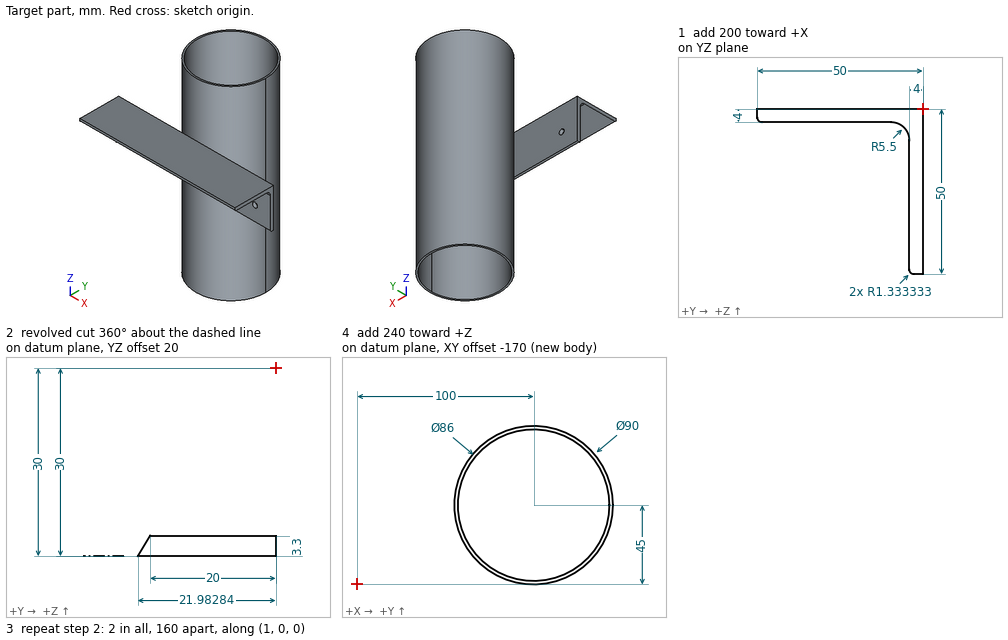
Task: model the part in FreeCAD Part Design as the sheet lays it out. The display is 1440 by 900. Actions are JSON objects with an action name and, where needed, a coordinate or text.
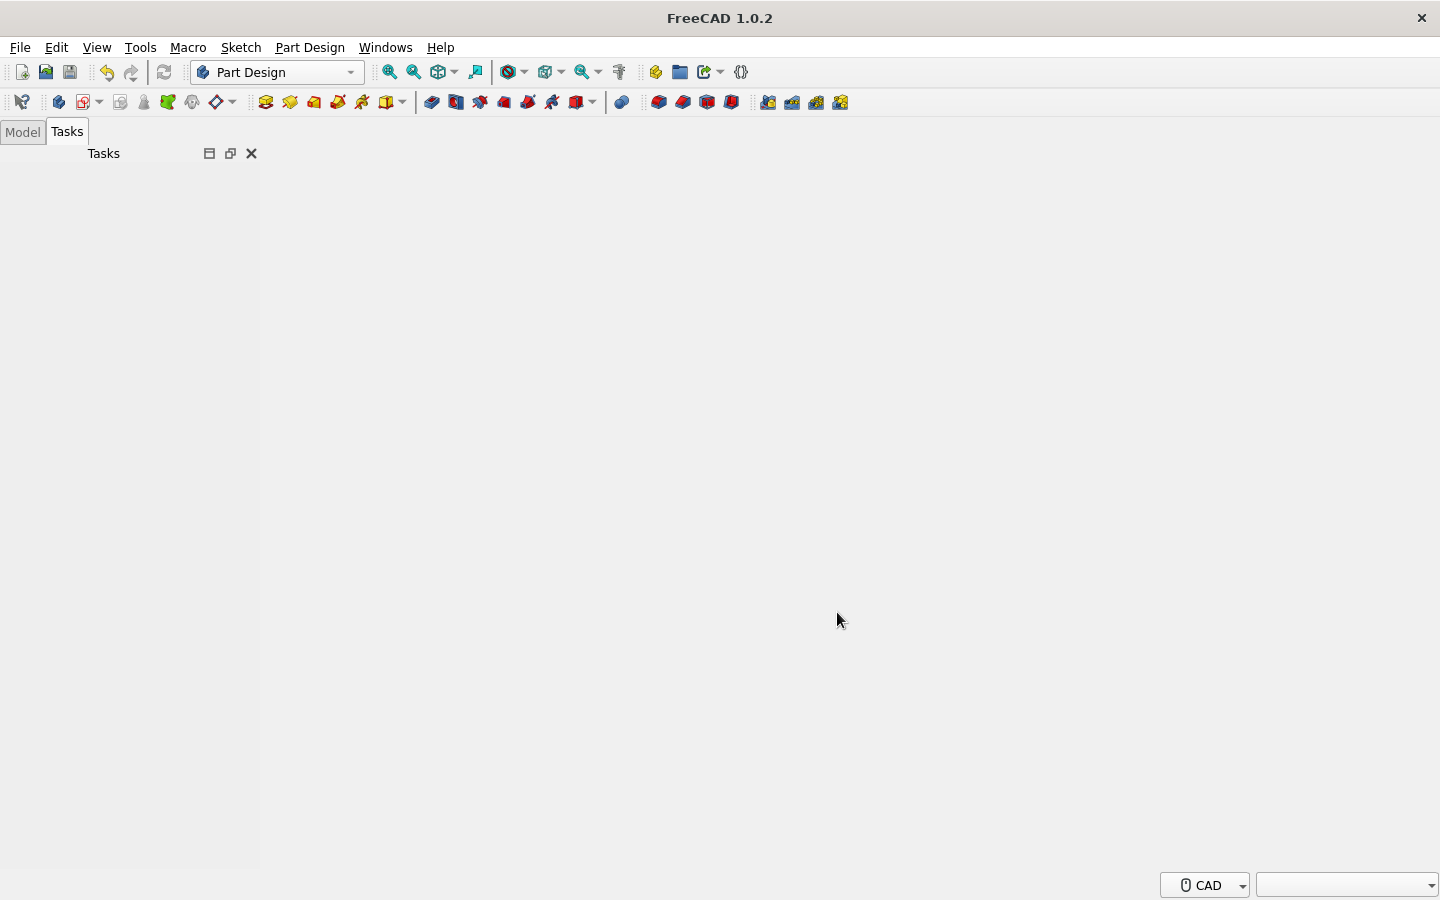
{"action": "left_click", "coordinate": [22, 72]}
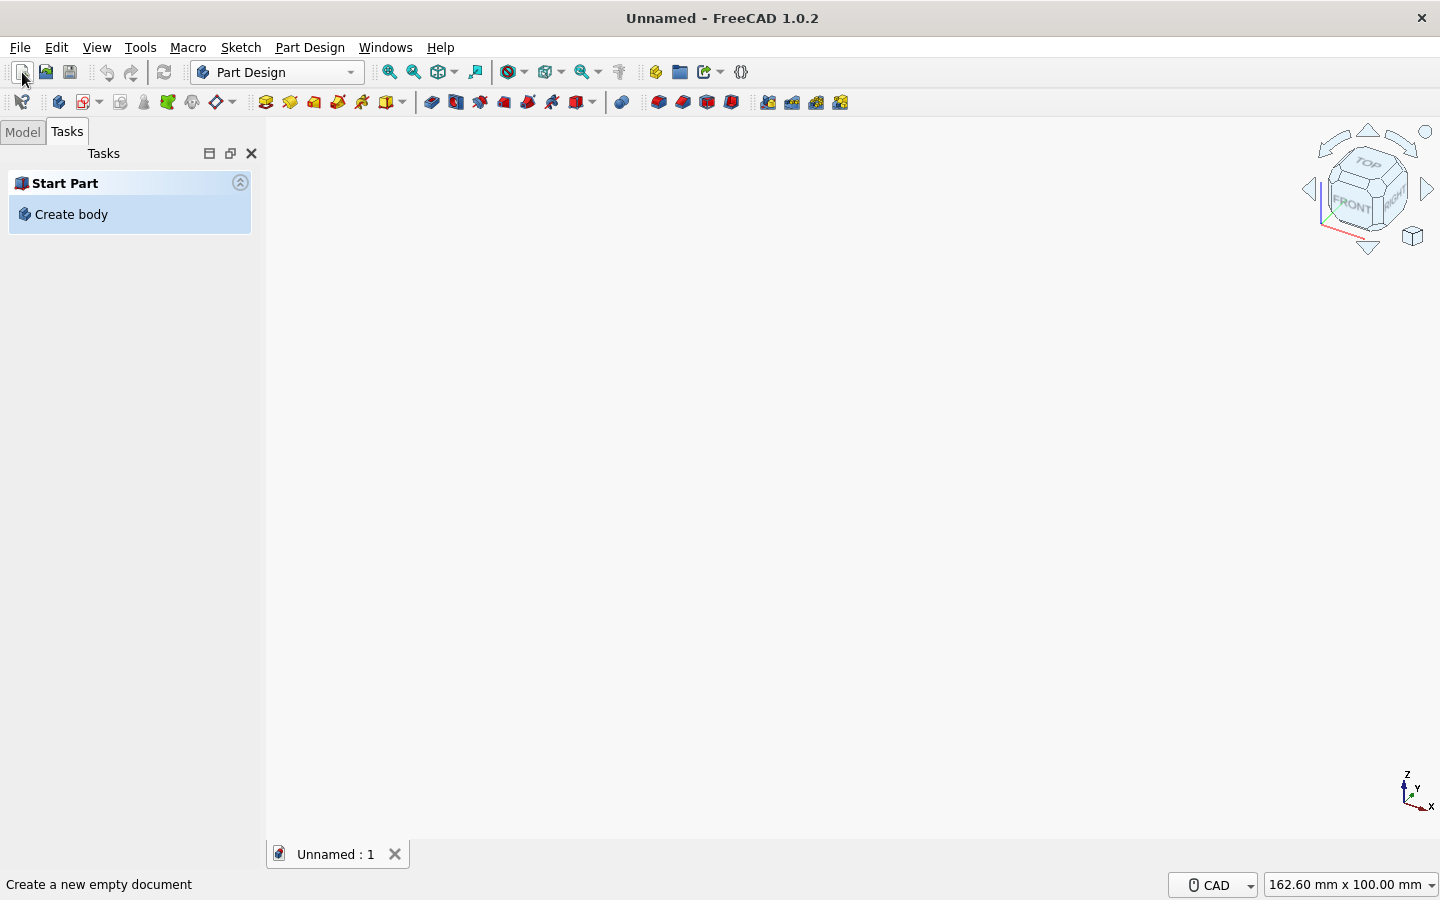
{"action": "left_click", "coordinate": [84, 102]}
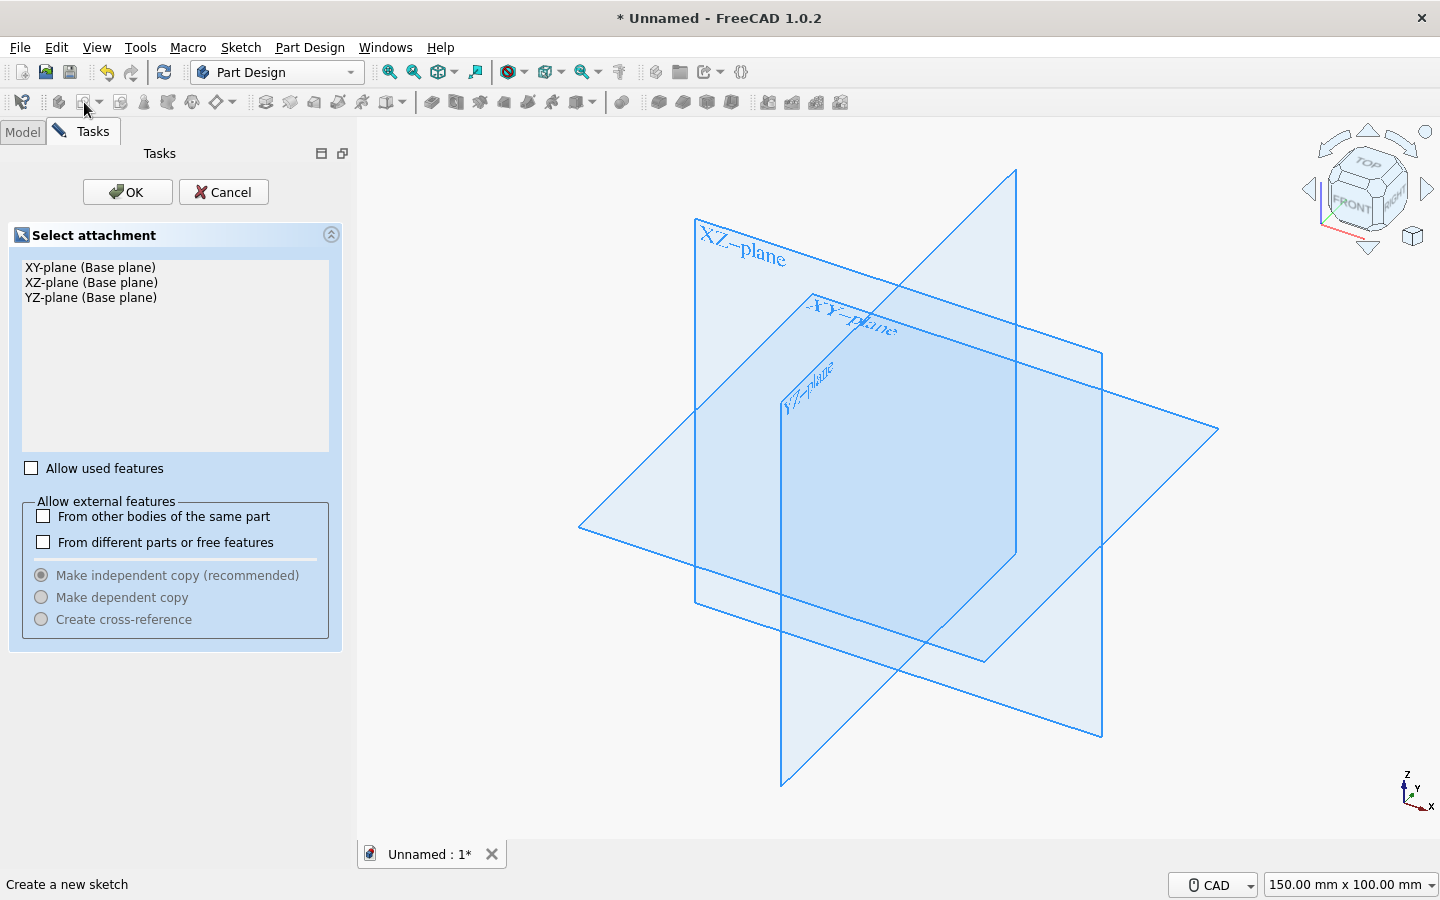
{"action": "left_click", "coordinate": [82, 298]}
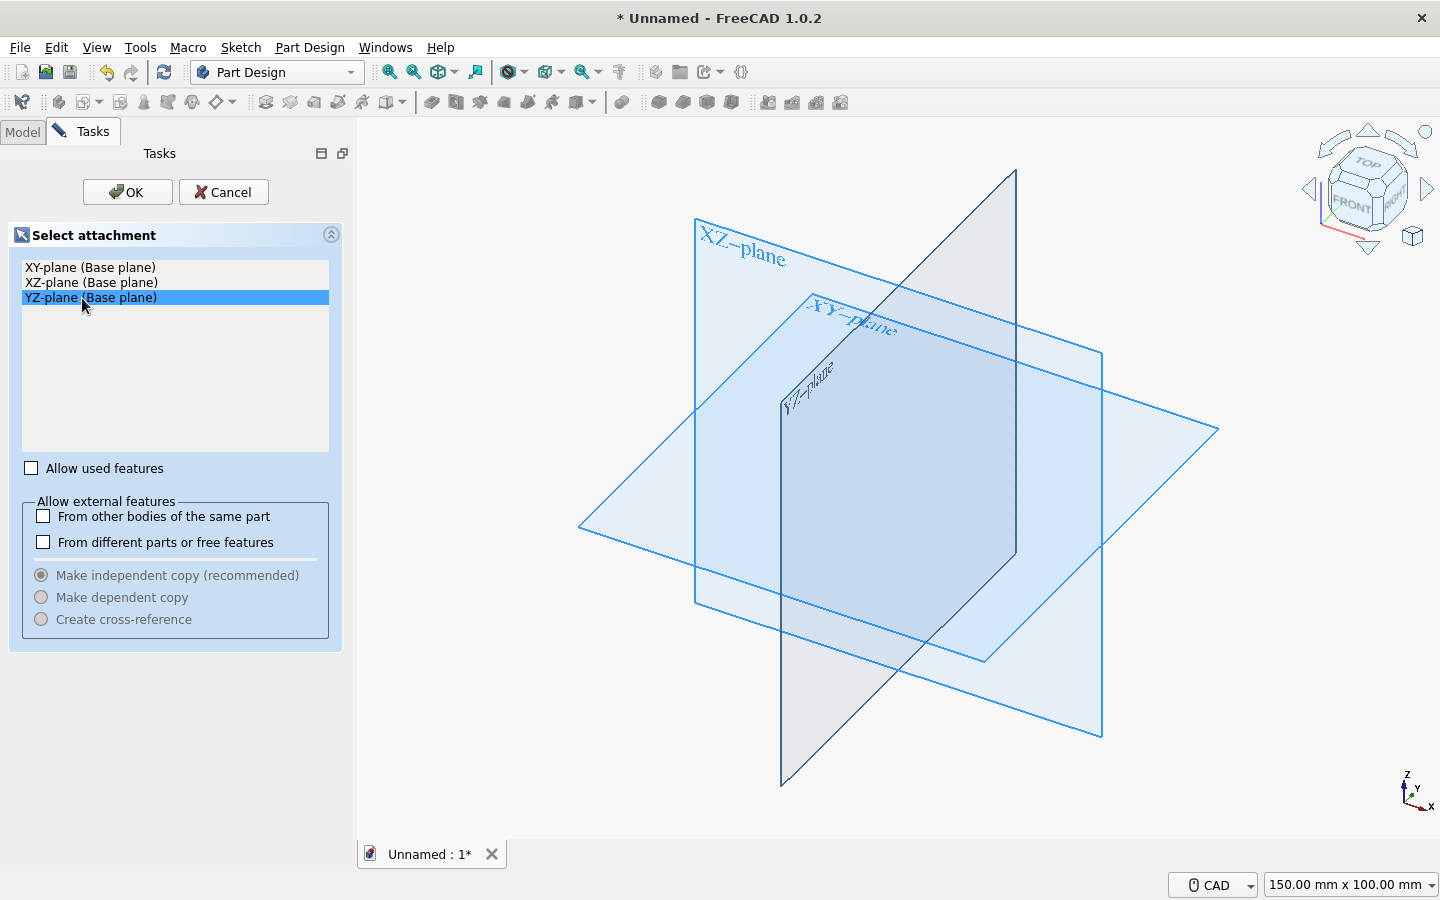
{"action": "left_click", "coordinate": [128, 192]}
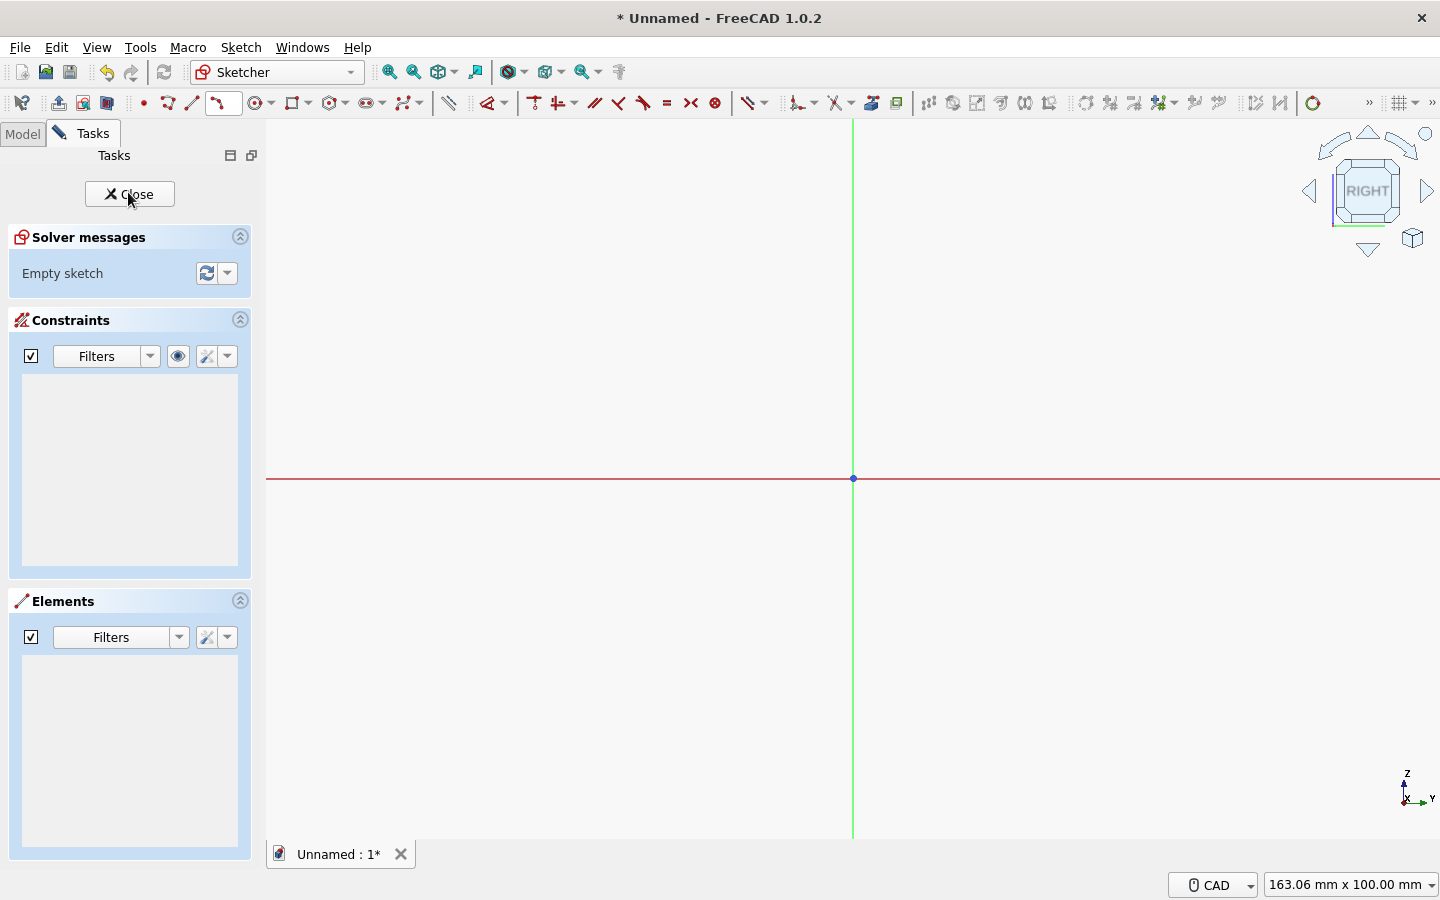
{"action": "scroll", "coordinate": [1275, 147], "scroll_direction": "down", "scroll_amount": 1}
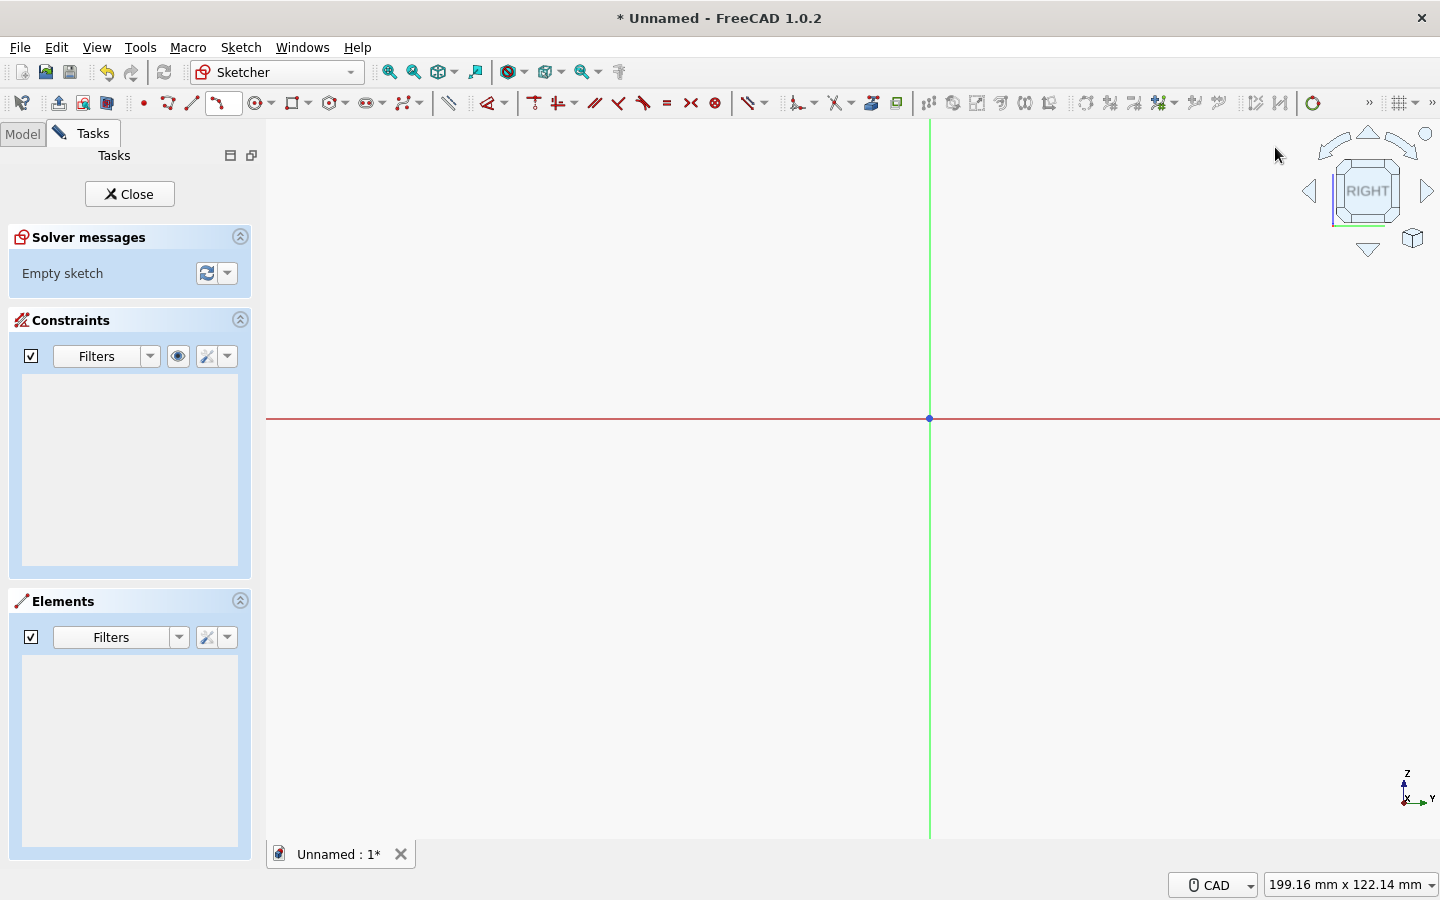
{"action": "scroll", "coordinate": [778, 743], "scroll_direction": "up", "scroll_amount": 2}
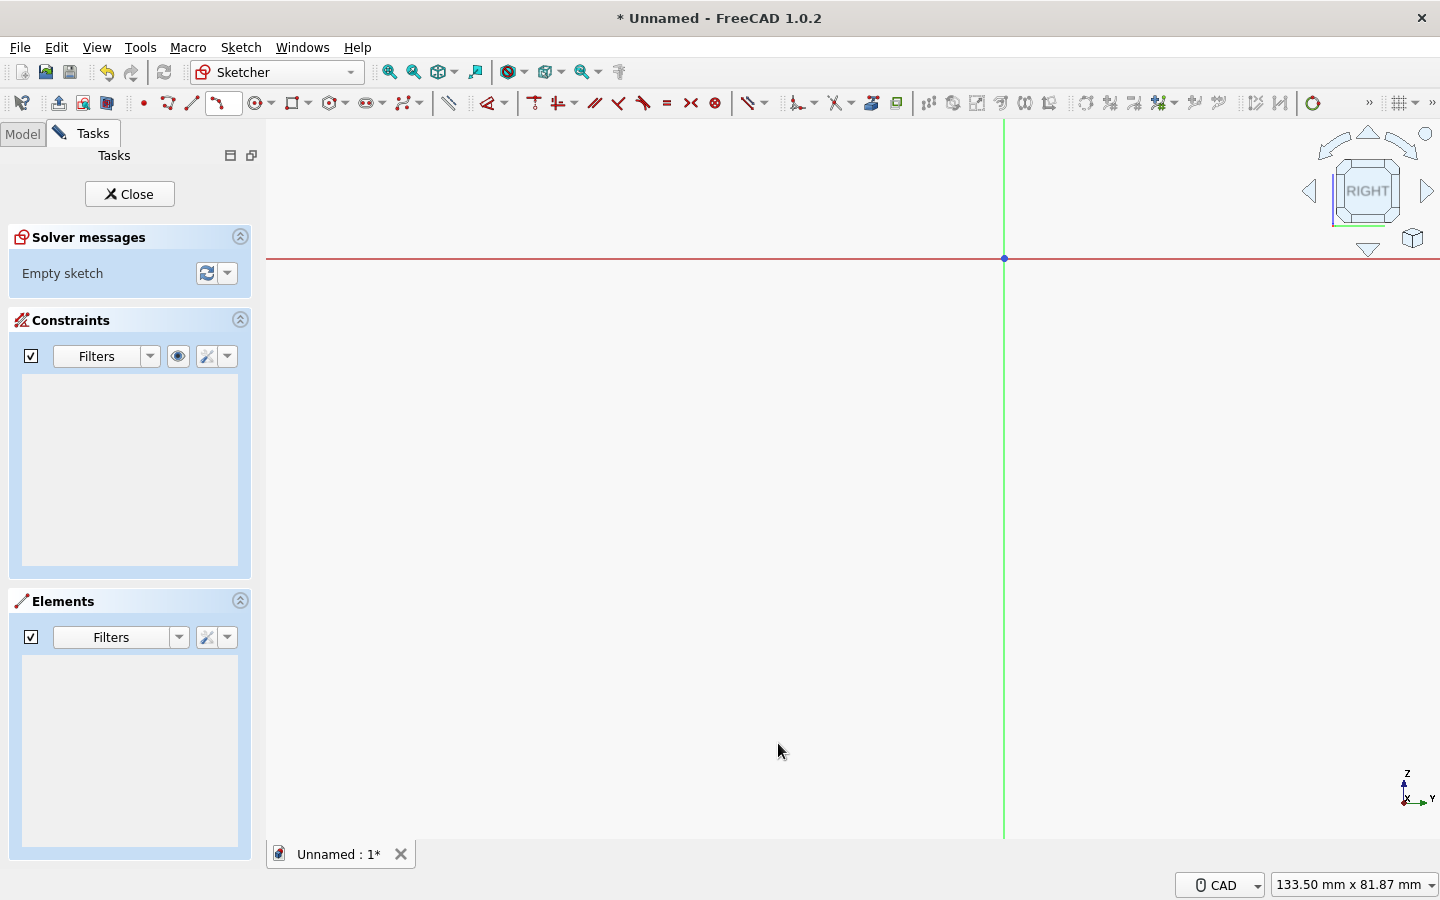
{"action": "left_click", "coordinate": [192, 104]}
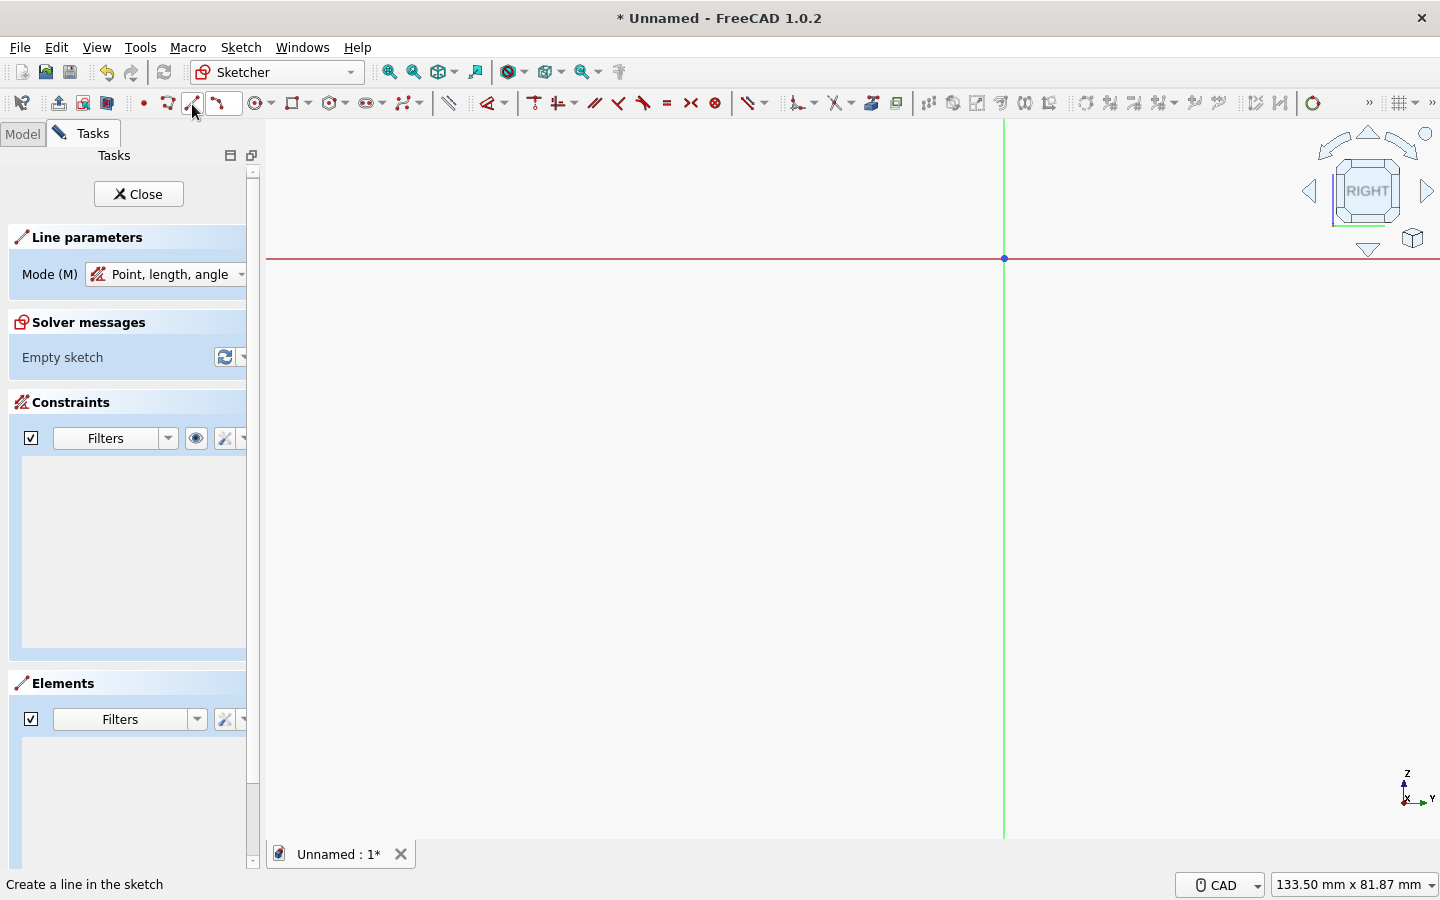
{"action": "left_click", "coordinate": [576, 294]}
{"action": "left_click", "coordinate": [920, 294]}